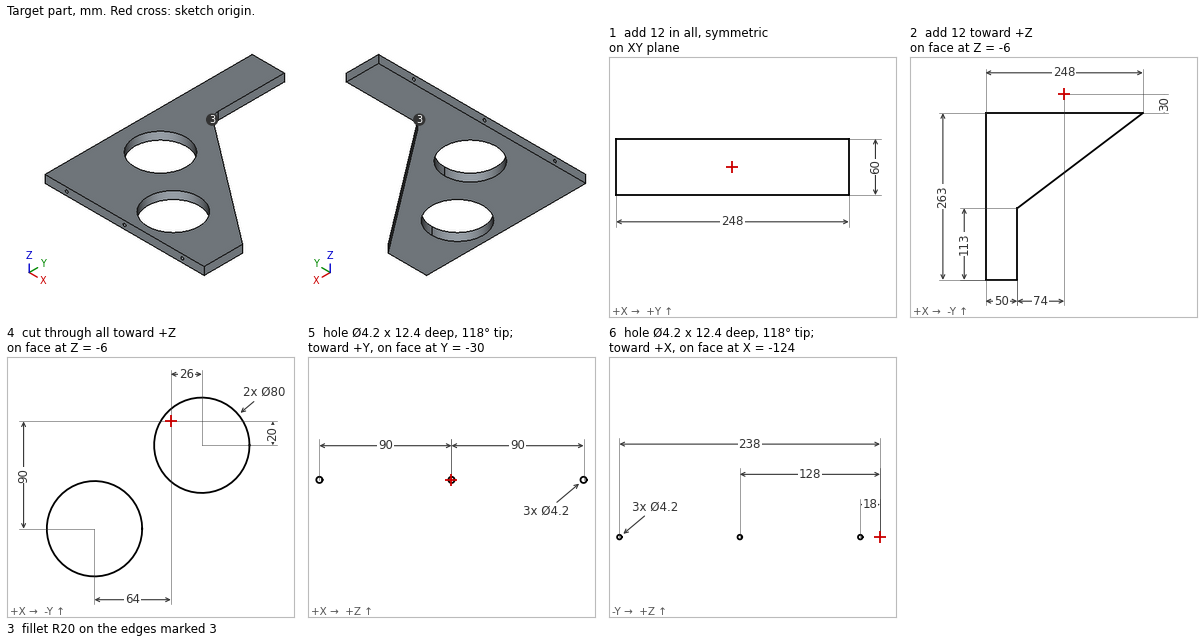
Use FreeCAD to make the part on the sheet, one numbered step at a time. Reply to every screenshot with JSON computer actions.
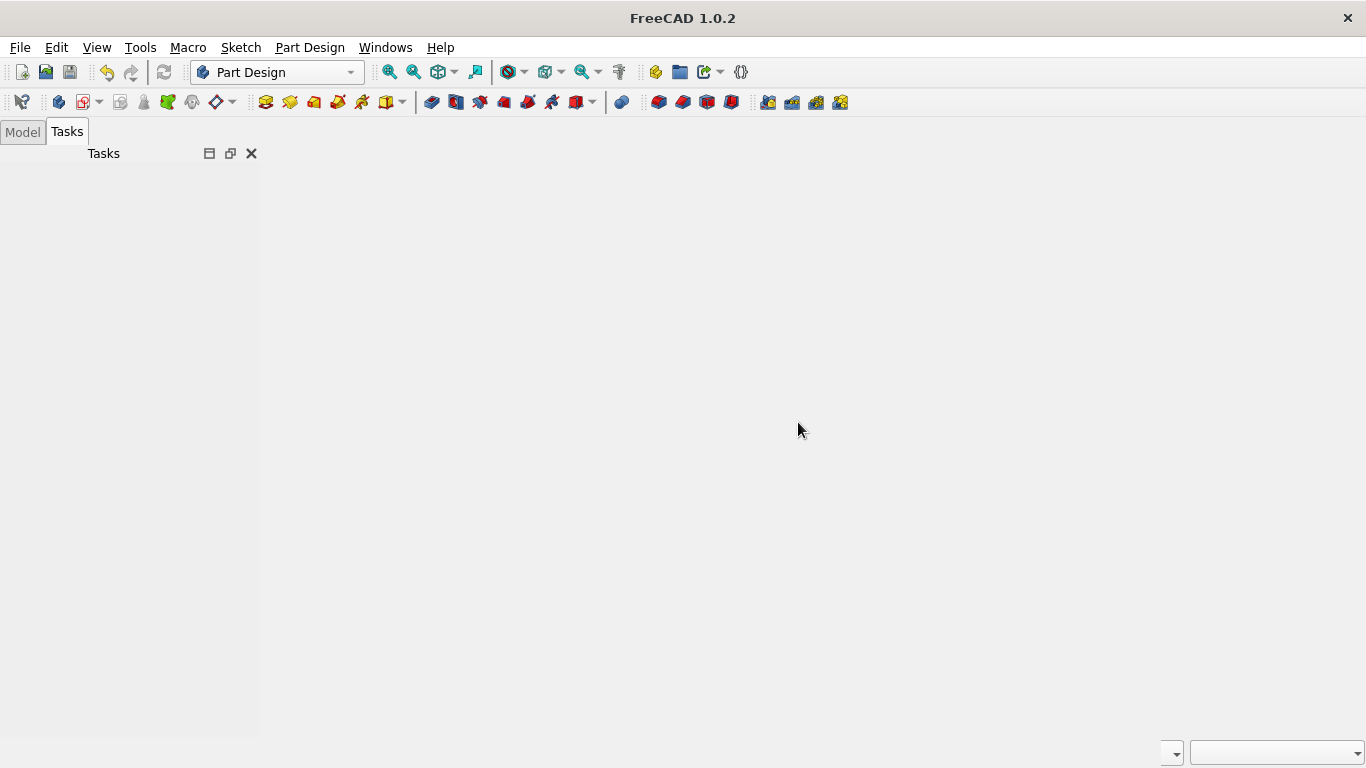
{"action": "left_click", "coordinate": [22, 72]}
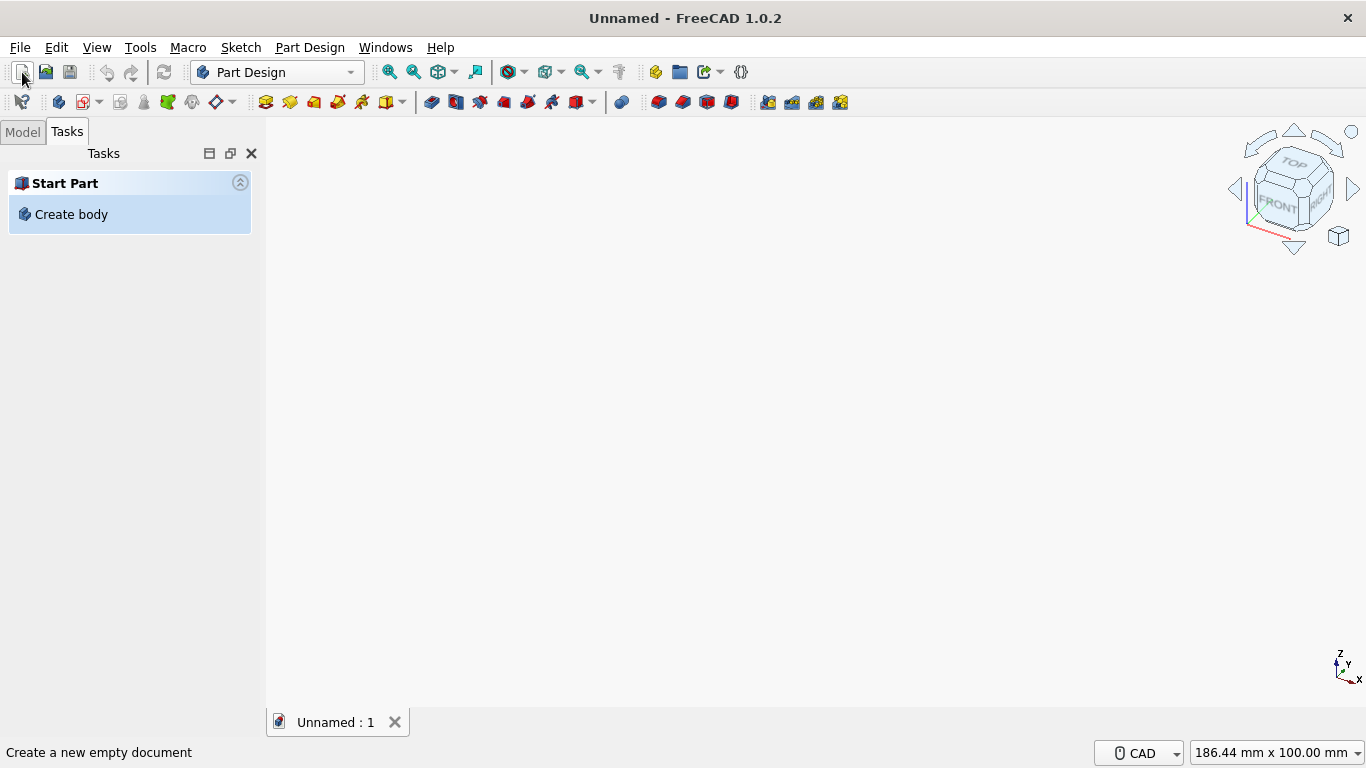
{"action": "left_click", "coordinate": [84, 102]}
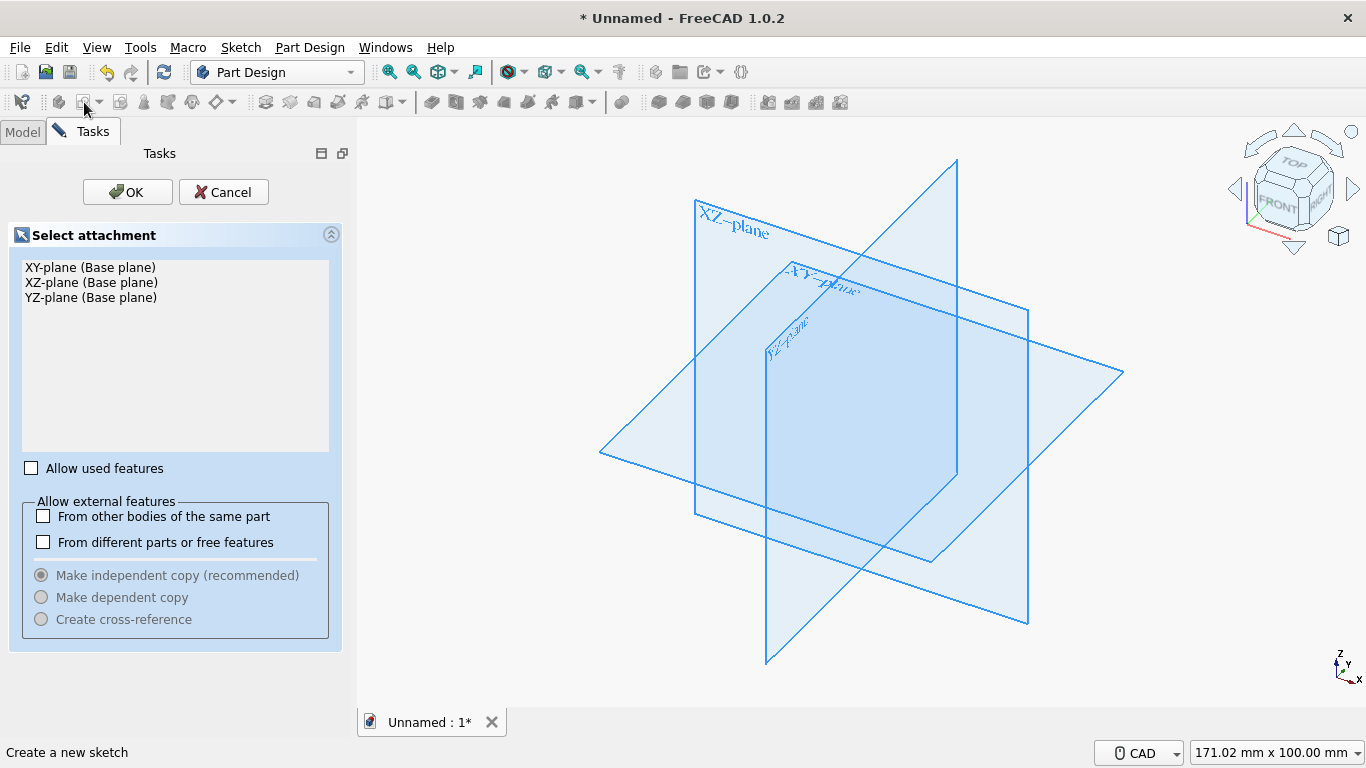
{"action": "left_click", "coordinate": [82, 268]}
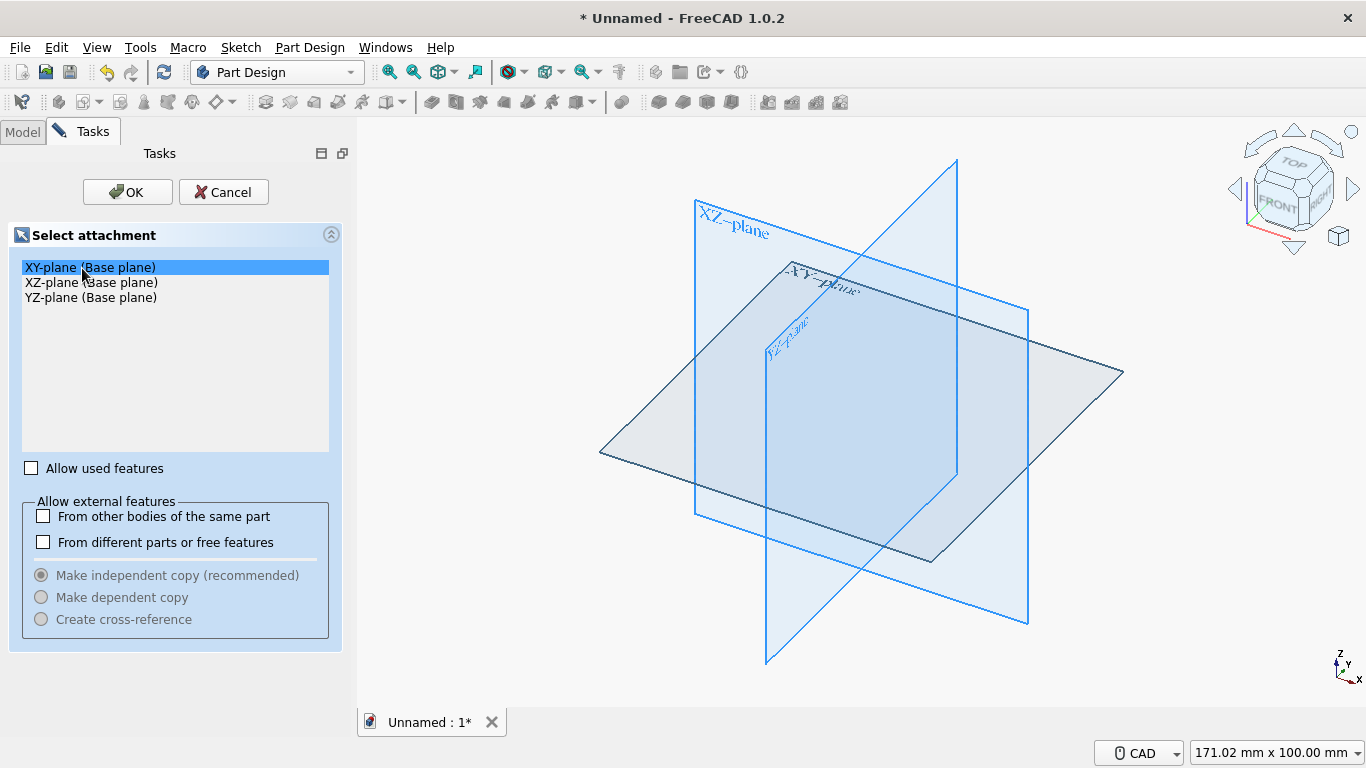
{"action": "left_click", "coordinate": [128, 192]}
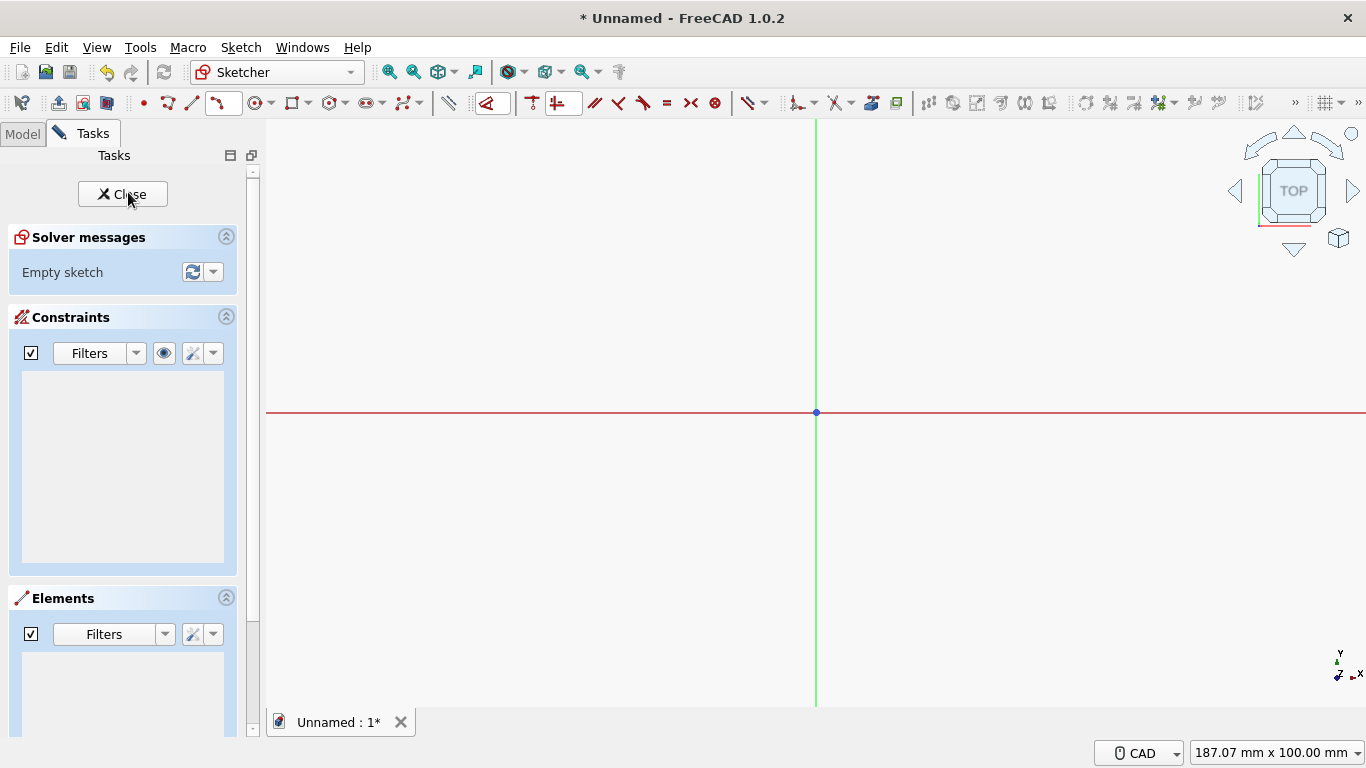
{"action": "scroll", "coordinate": [692, 413], "scroll_direction": "down", "scroll_amount": 4}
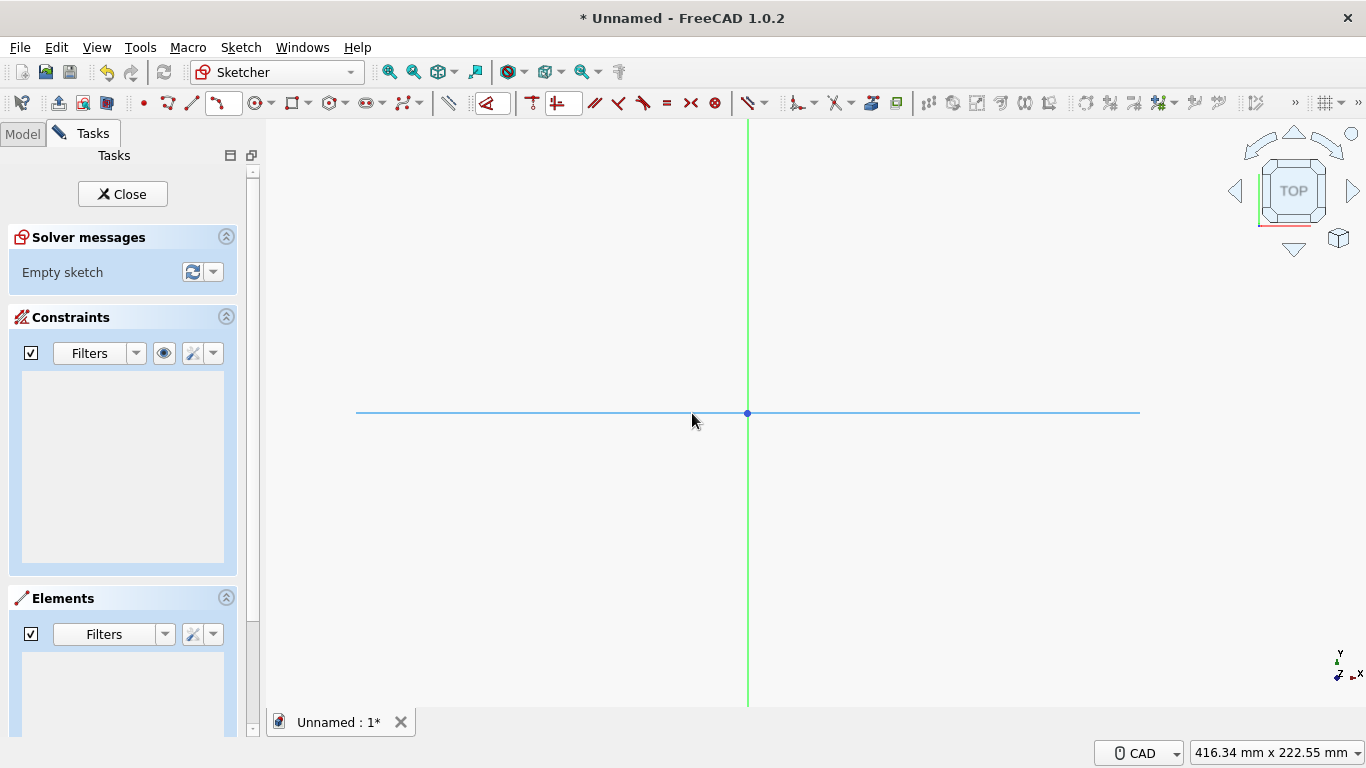
{"action": "key", "text": "g v"}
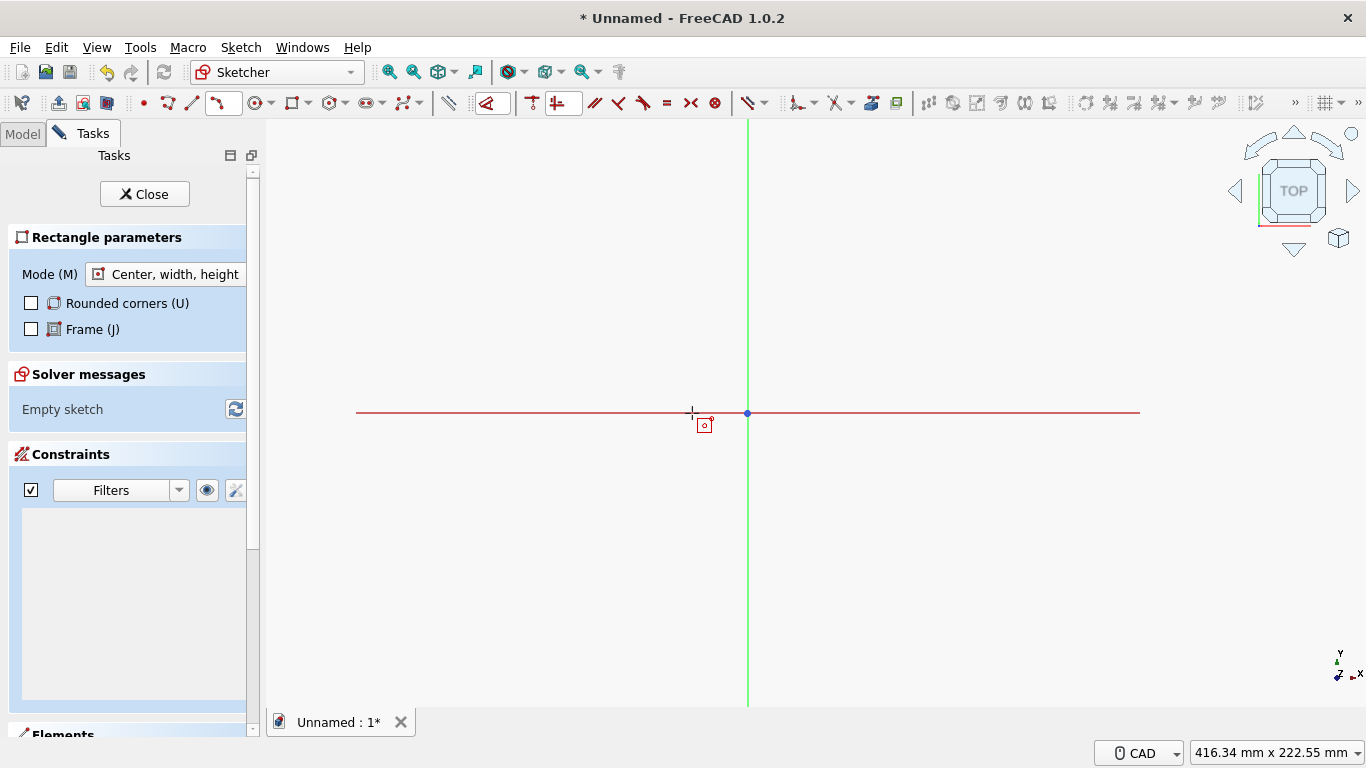
{"action": "left_click", "coordinate": [748, 413]}
{"action": "mouse_move", "coordinate": [1076, 334]}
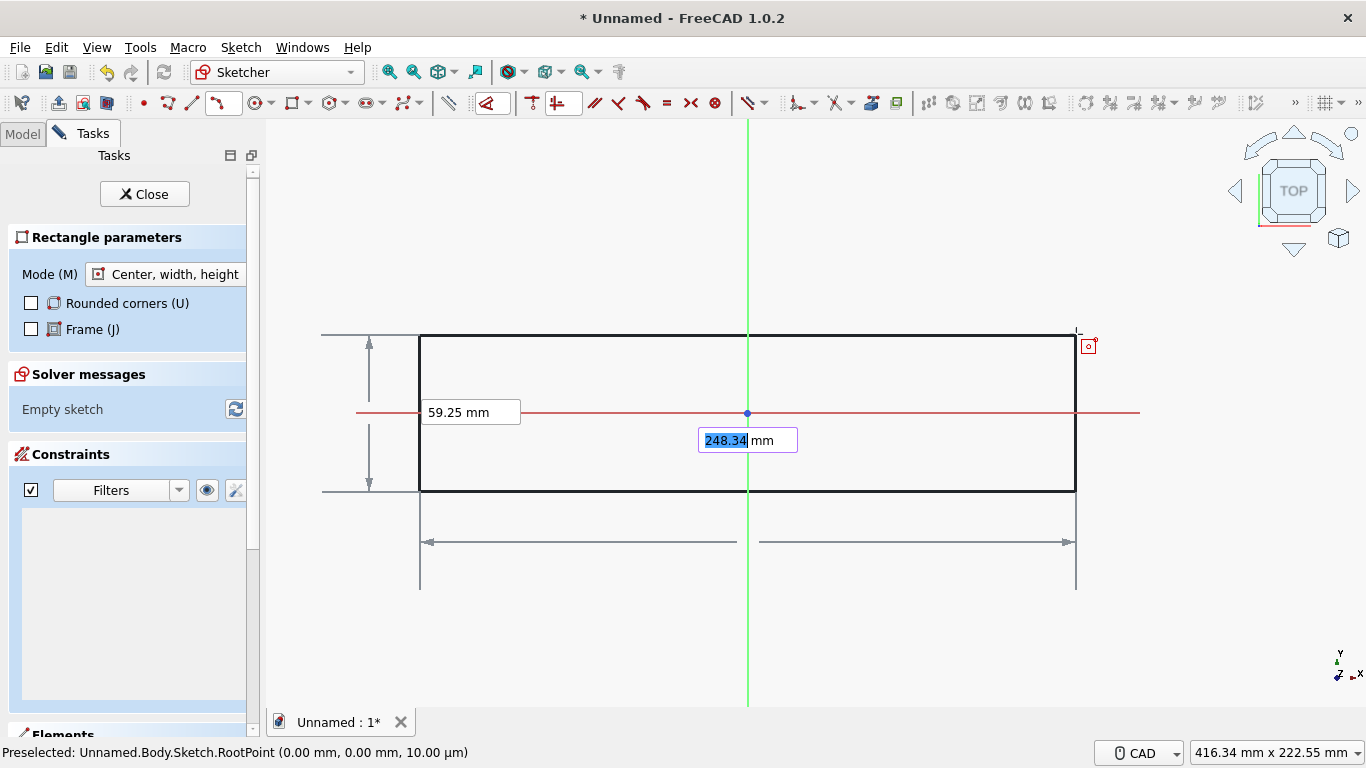
{"action": "type", "text": "248"}
{"action": "key", "text": "Tab"}
{"action": "type", "text": "60"}
{"action": "key", "text": "Return"}
{"action": "key", "text": "Escape"}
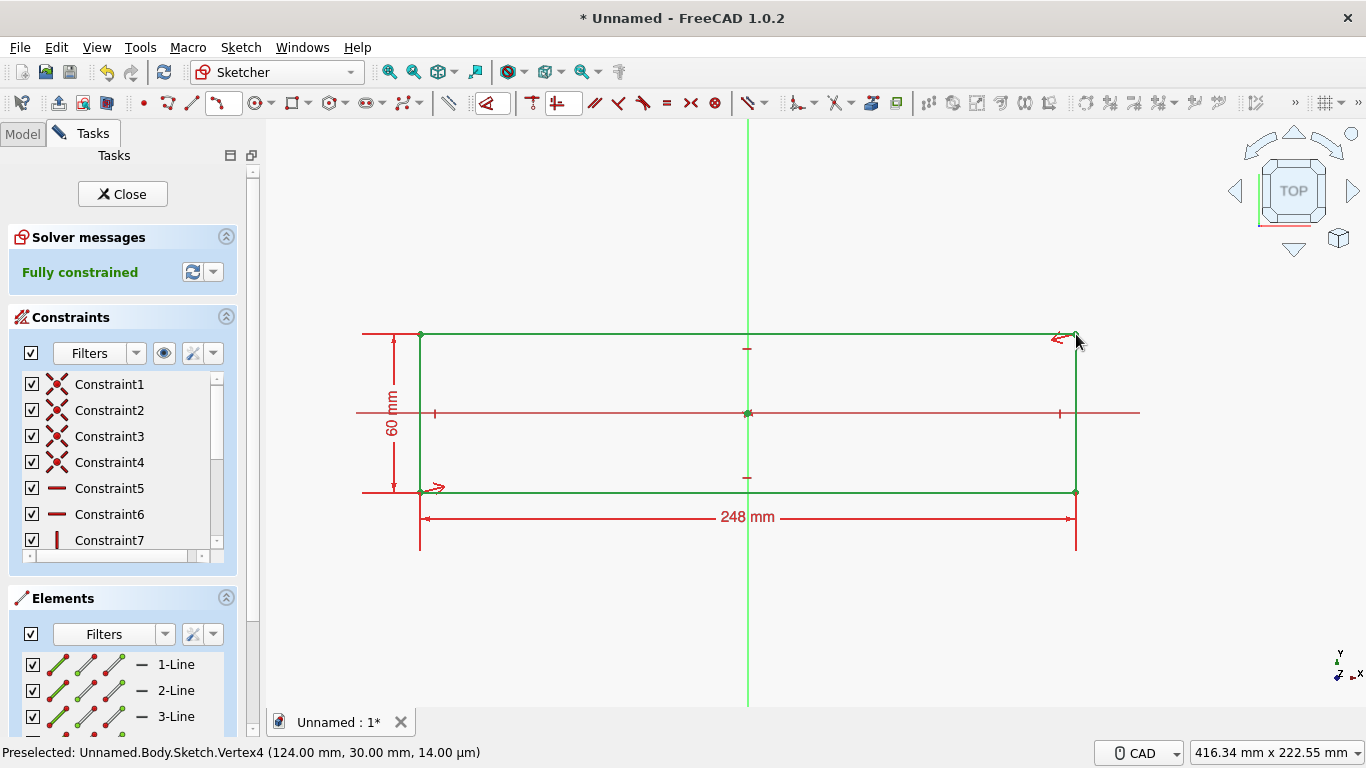
{"action": "left_click", "coordinate": [123, 194]}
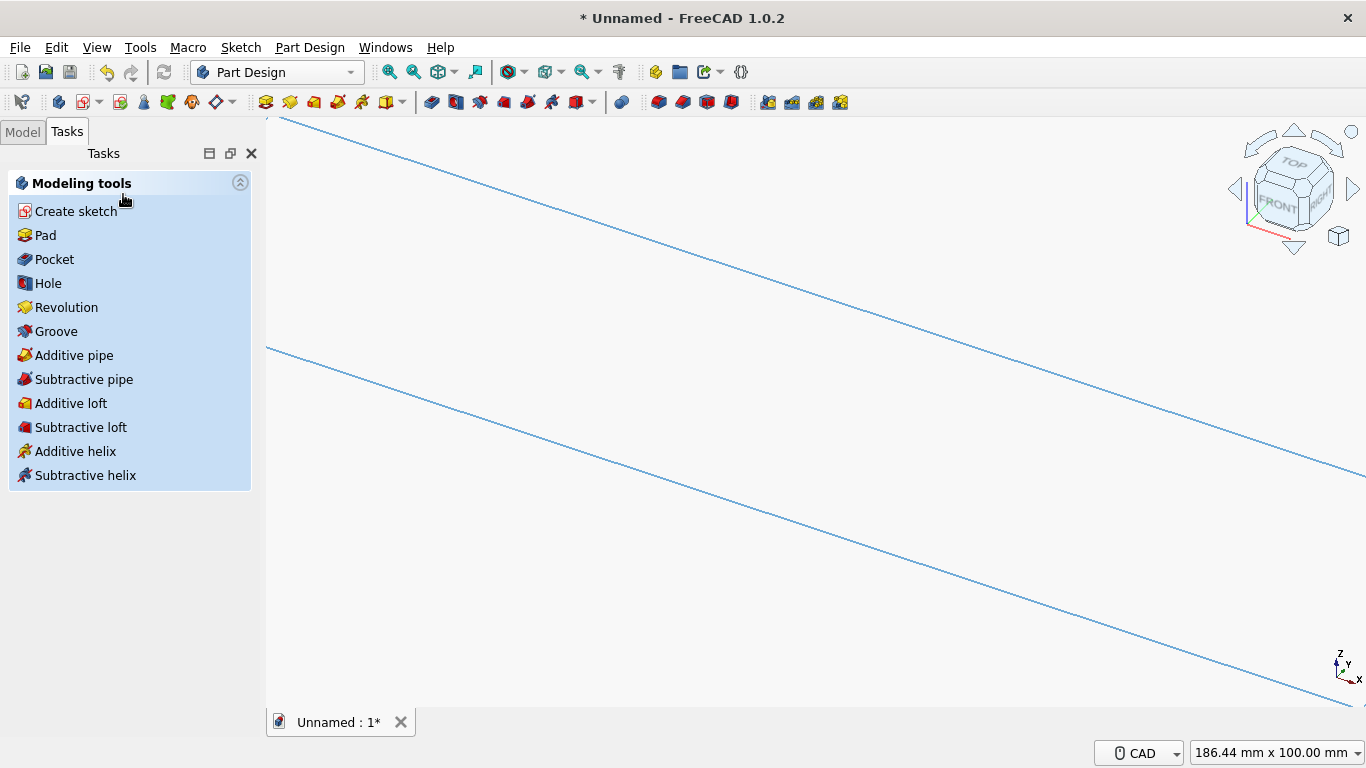
{"action": "left_click", "coordinate": [266, 102]}